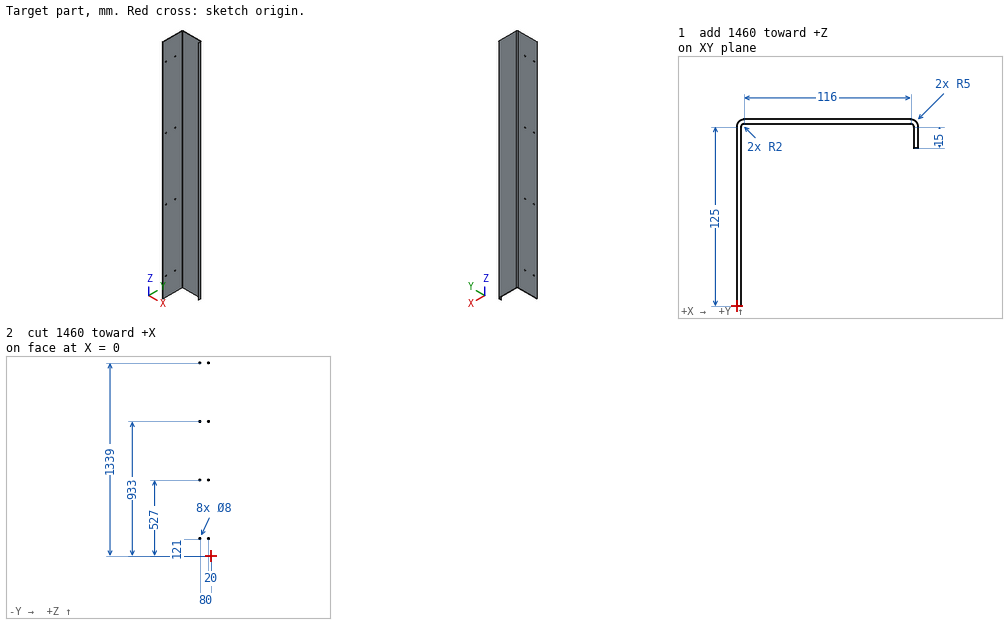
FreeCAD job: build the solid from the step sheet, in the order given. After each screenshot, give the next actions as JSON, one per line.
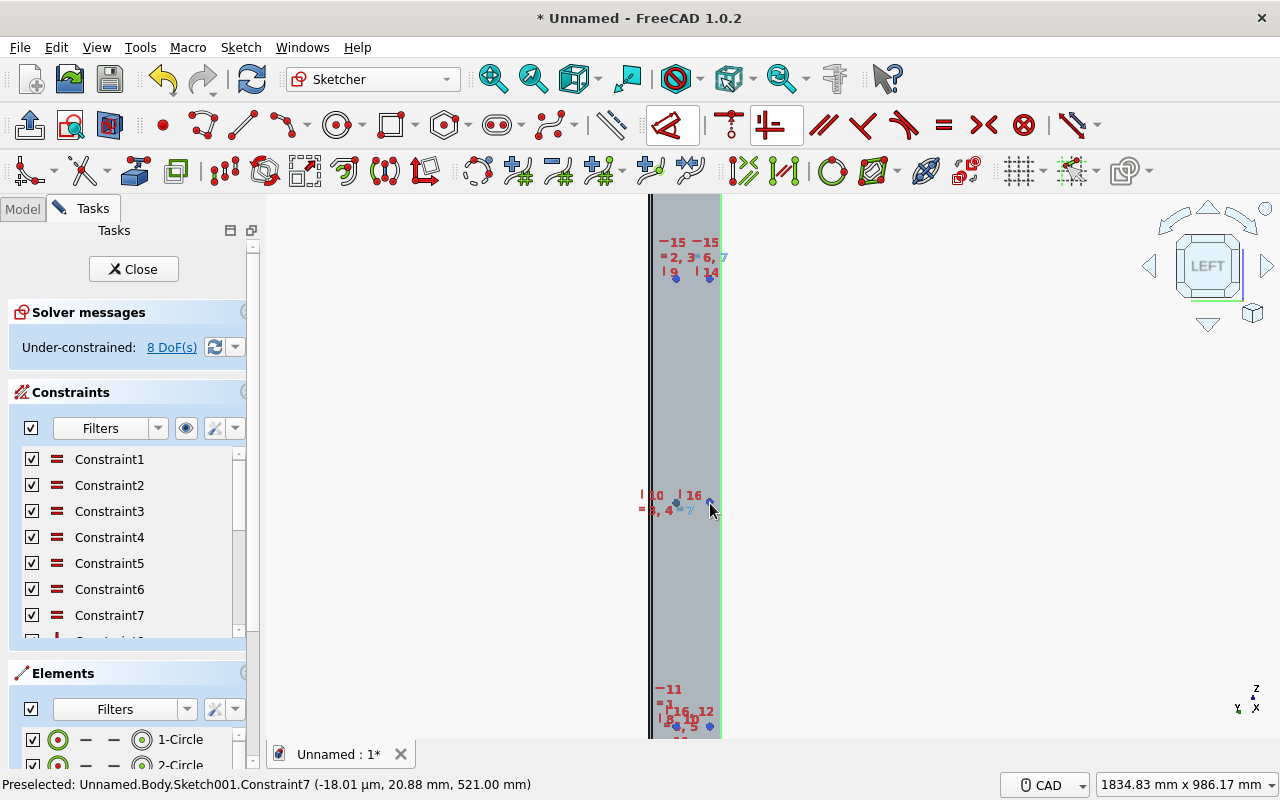
{"action": "left_click", "coordinate": [710, 502]}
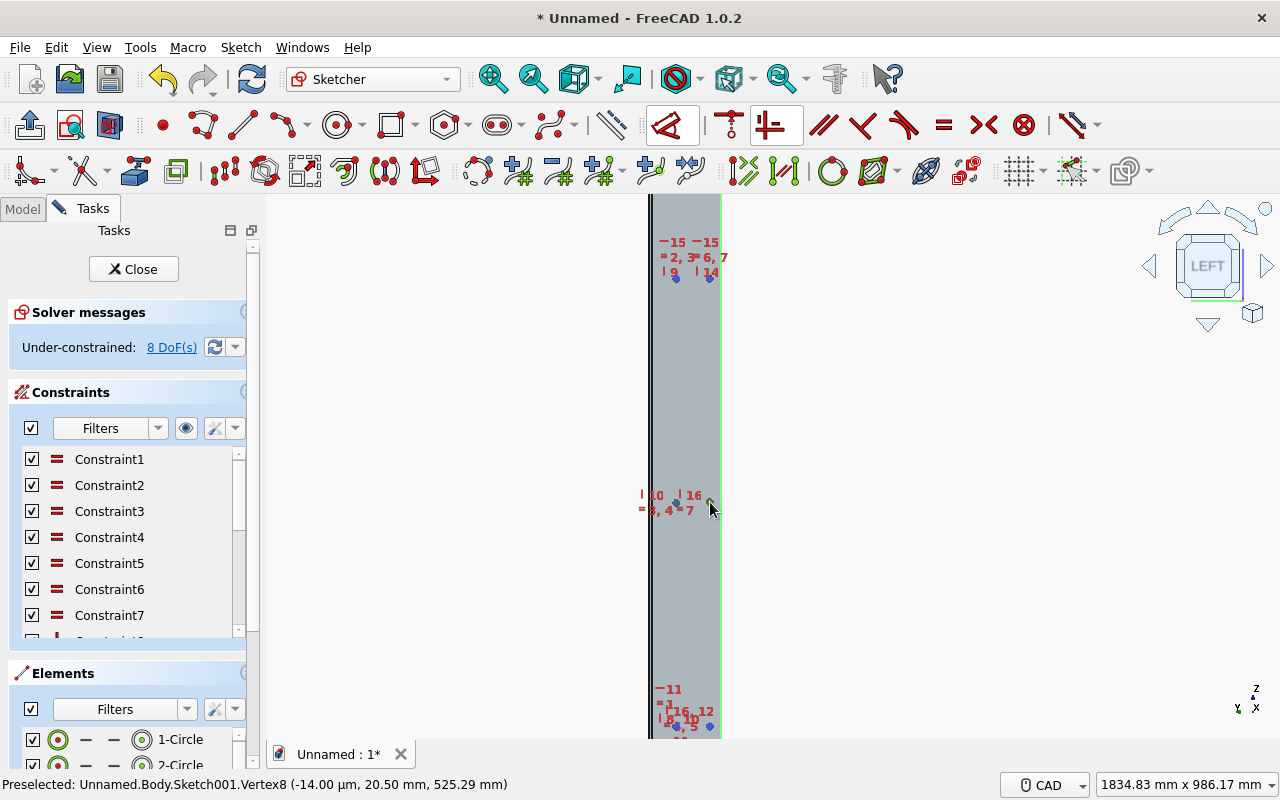
{"action": "left_click", "coordinate": [798, 126]}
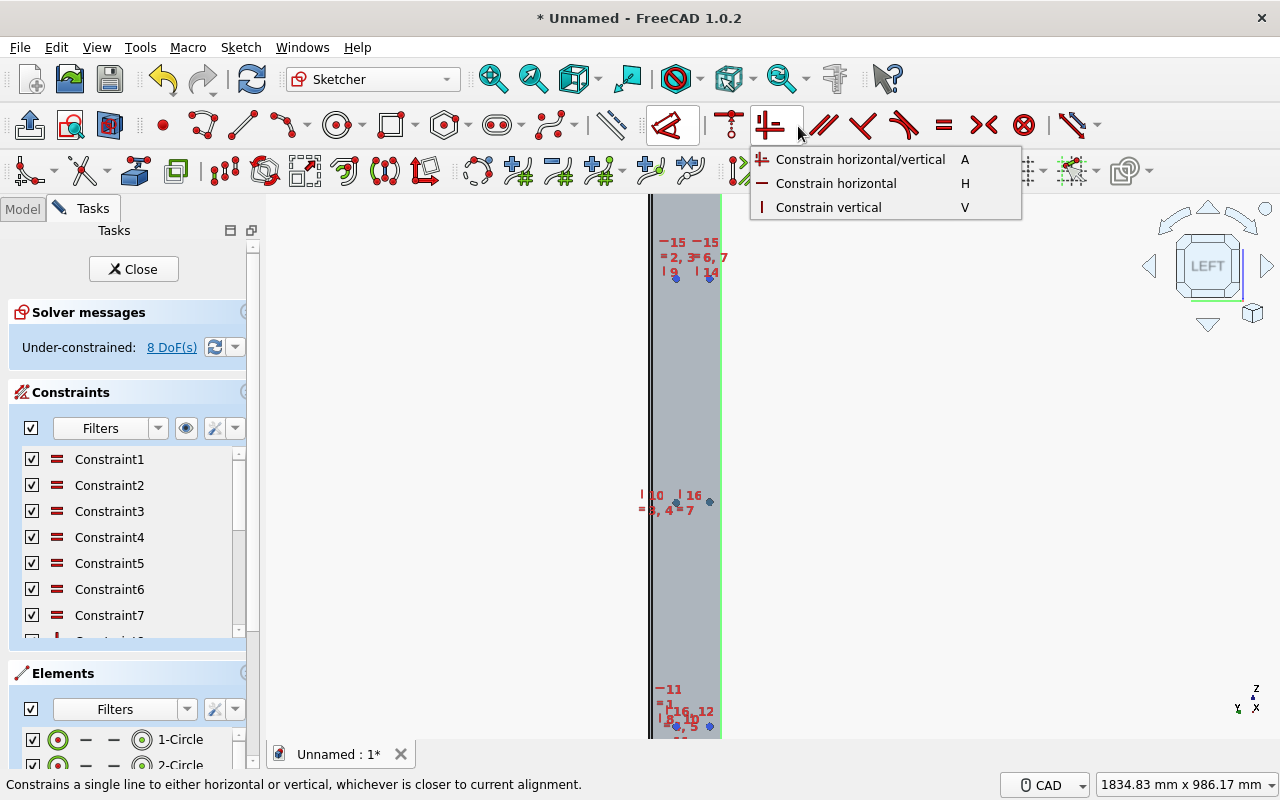
{"action": "left_click", "coordinate": [886, 183]}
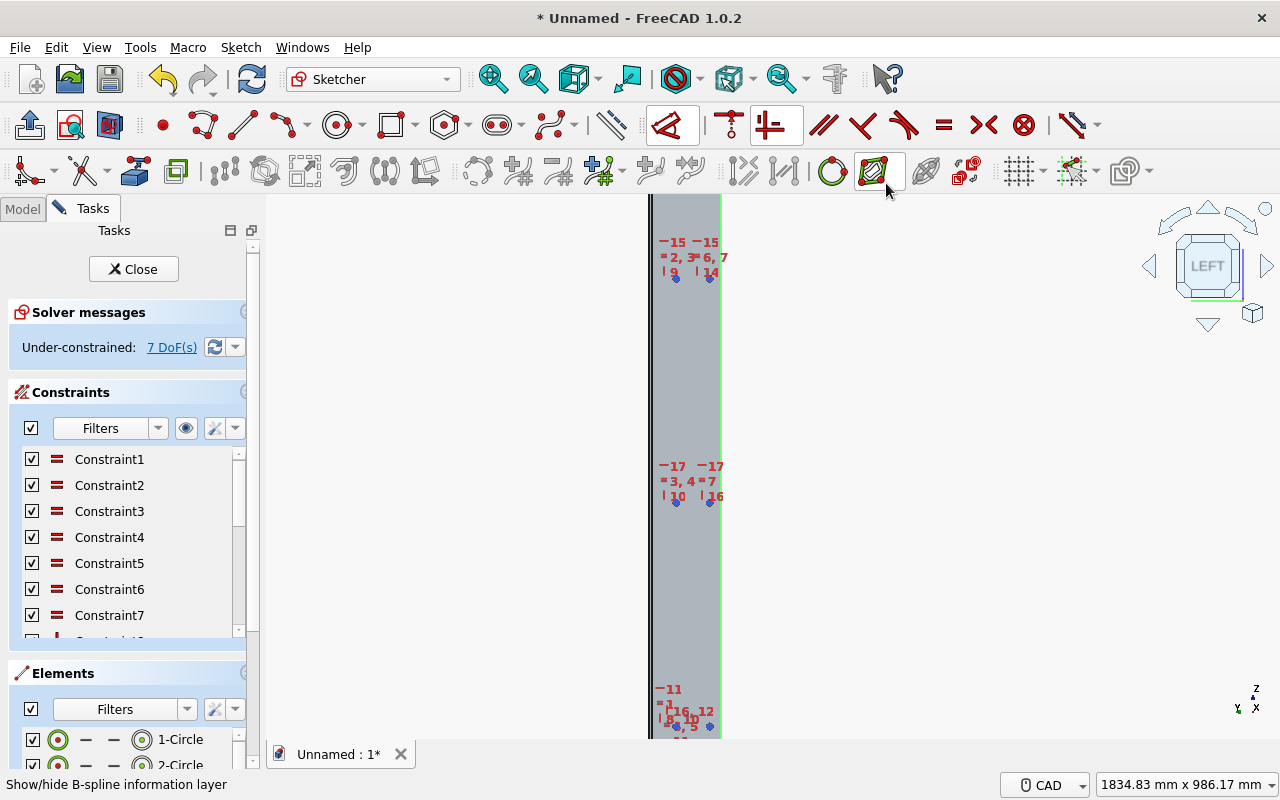
{"action": "scroll", "coordinate": [710, 503], "scroll_direction": "down", "scroll_amount": 4}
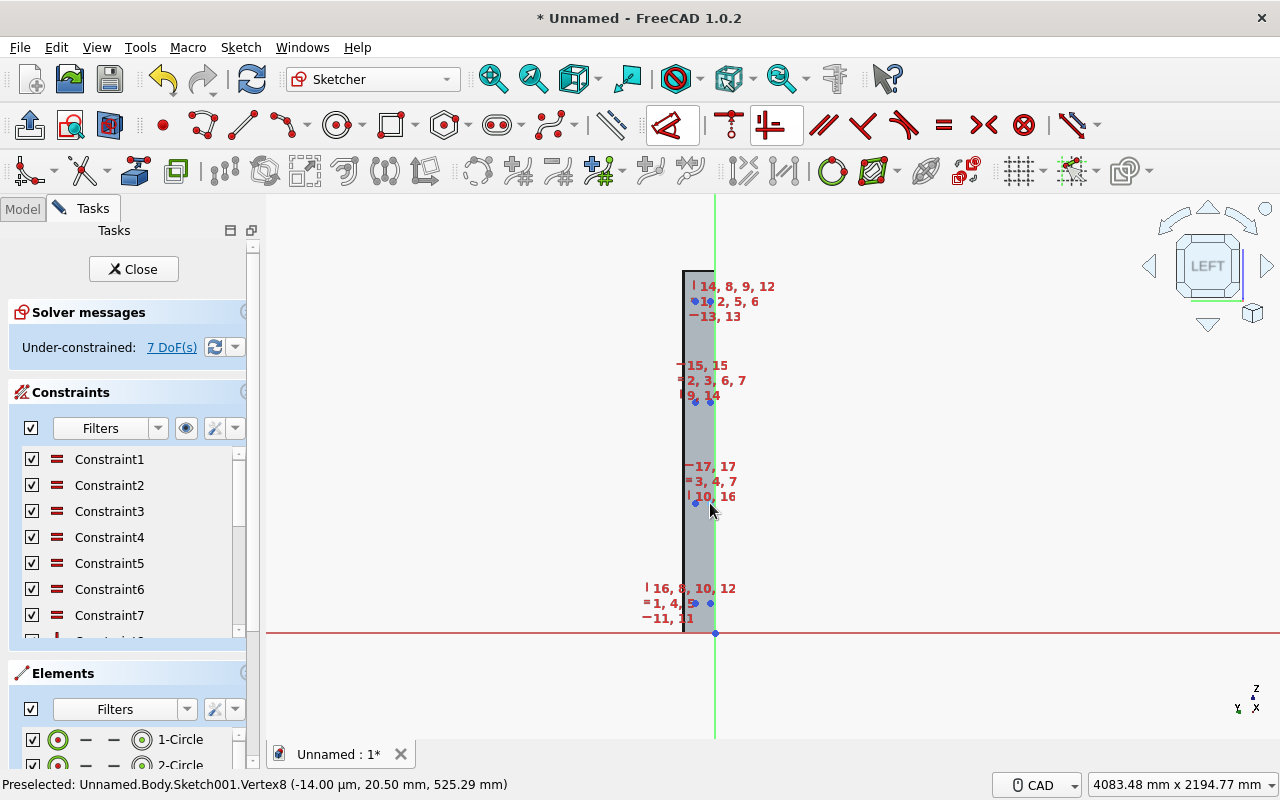
{"action": "scroll", "coordinate": [695, 602], "scroll_direction": "up", "scroll_amount": 15}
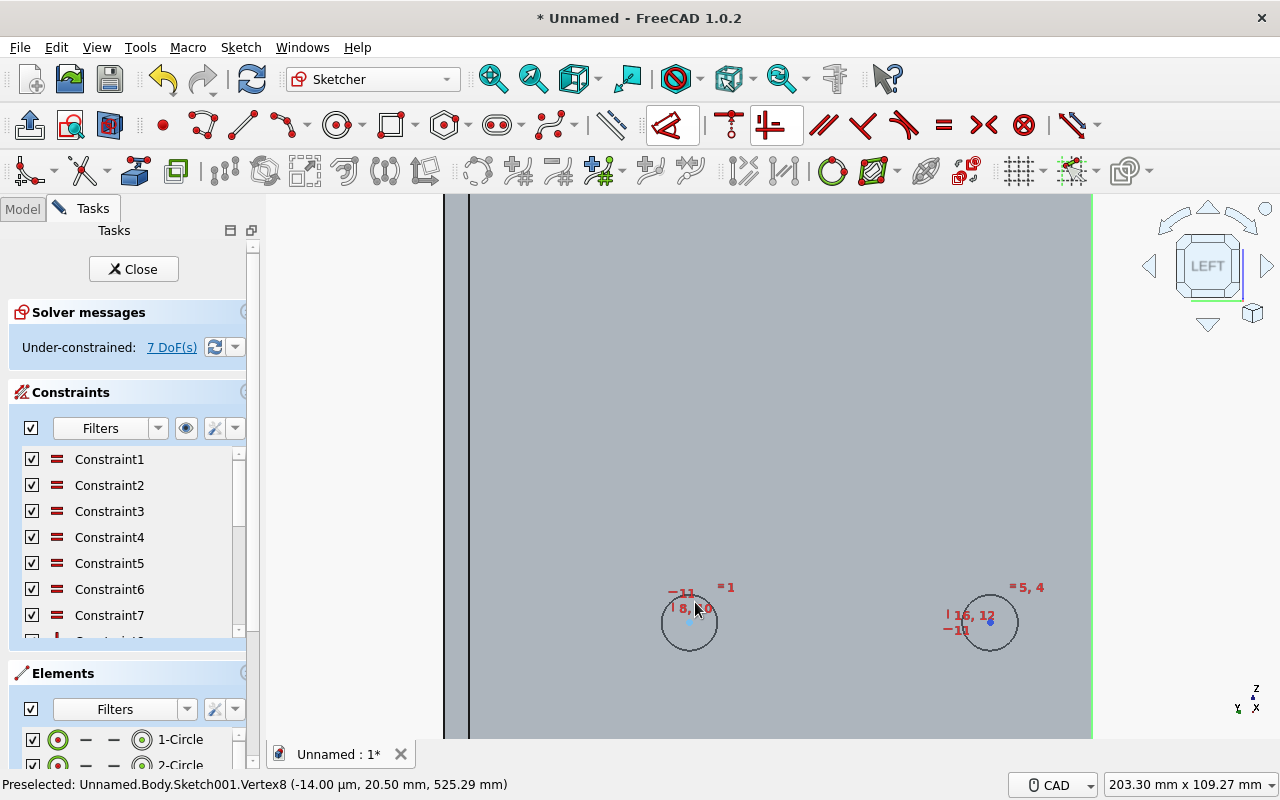
{"action": "left_click", "coordinate": [662, 622]}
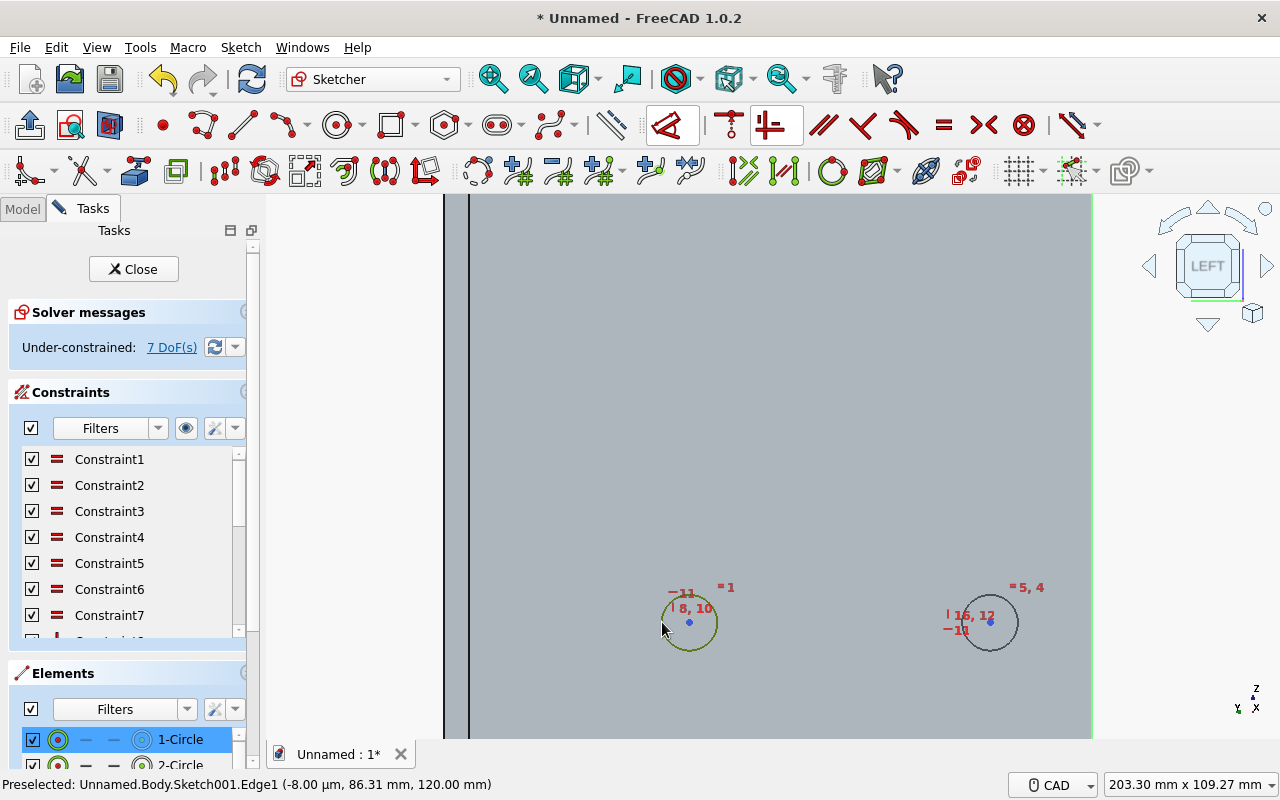
{"action": "key", "text": "k o"}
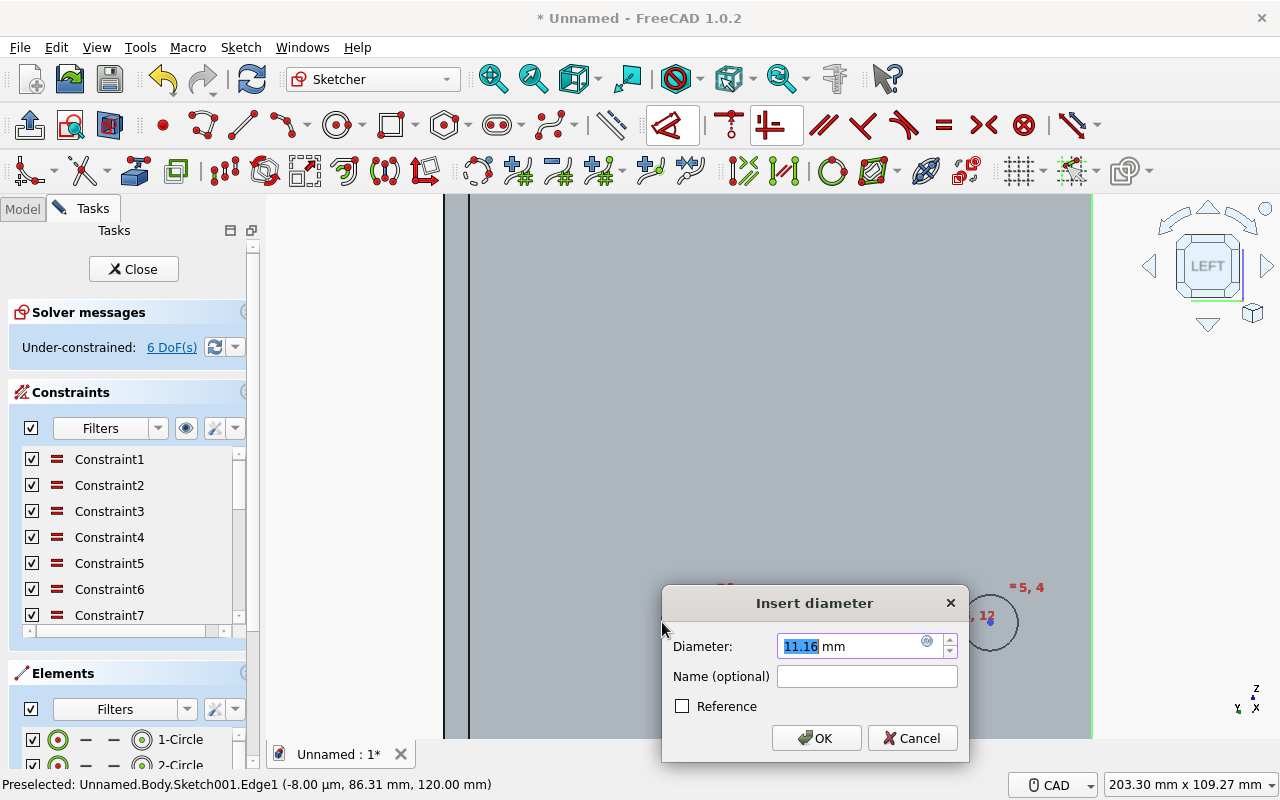
{"action": "type", "text": "8"}
{"action": "key", "text": "Return"}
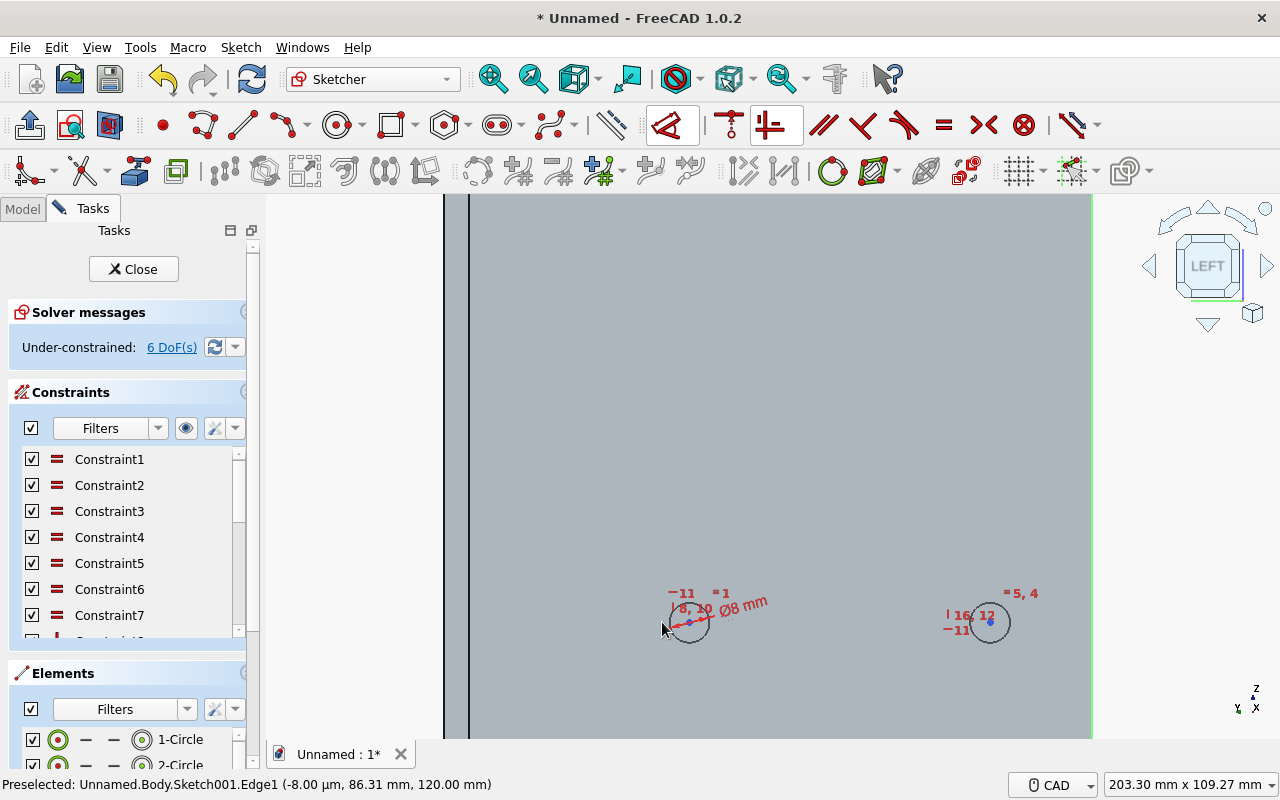
{"action": "scroll", "coordinate": [695, 603], "scroll_direction": "down", "scroll_amount": 15}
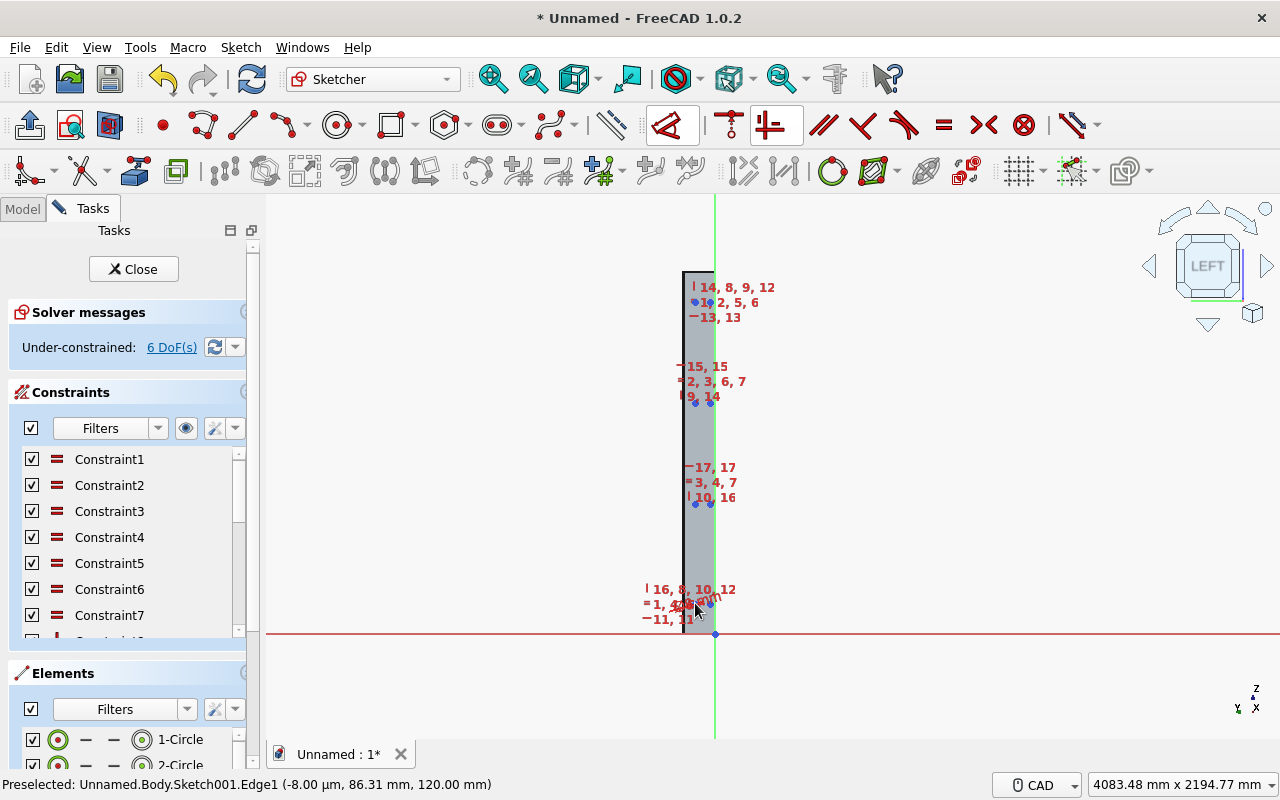
{"action": "scroll", "coordinate": [695, 605], "scroll_direction": "up", "scroll_amount": 4}